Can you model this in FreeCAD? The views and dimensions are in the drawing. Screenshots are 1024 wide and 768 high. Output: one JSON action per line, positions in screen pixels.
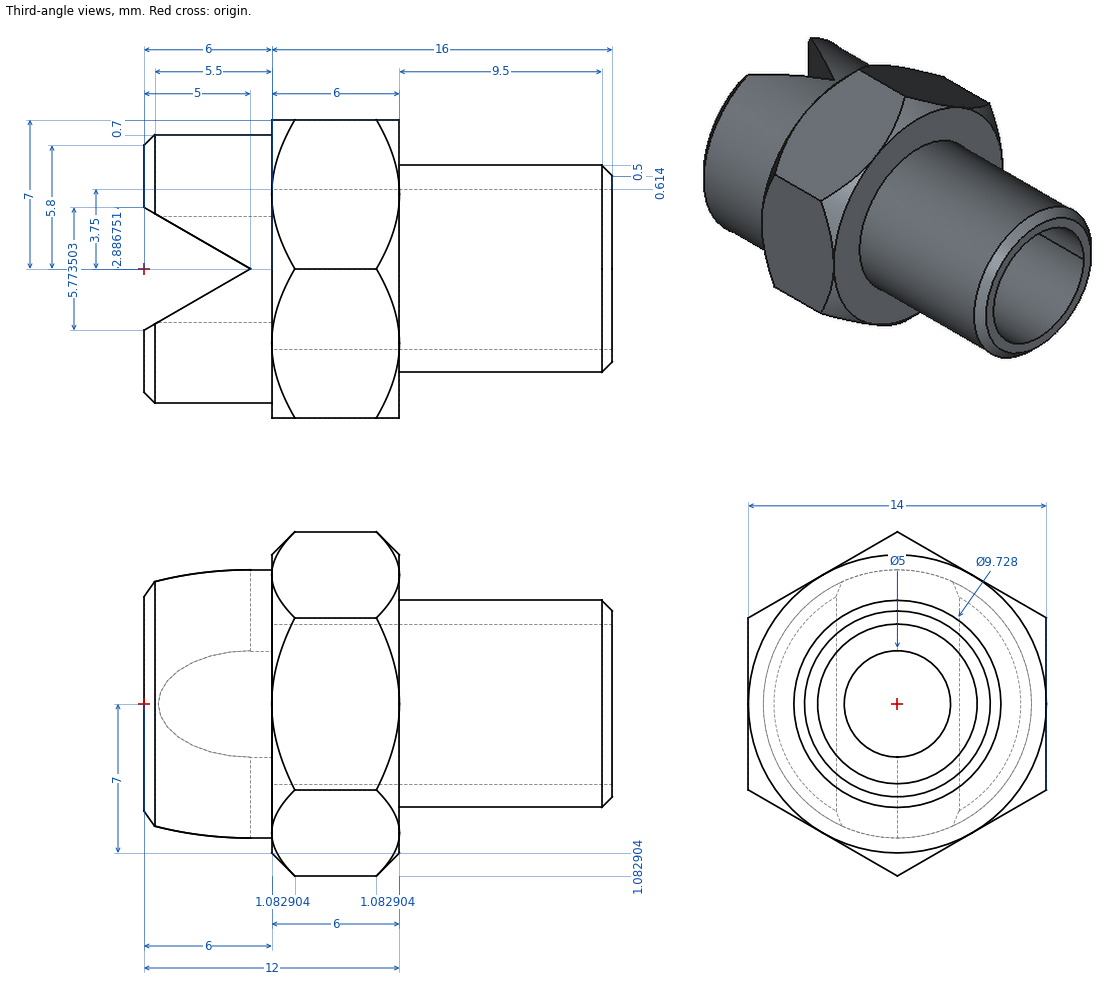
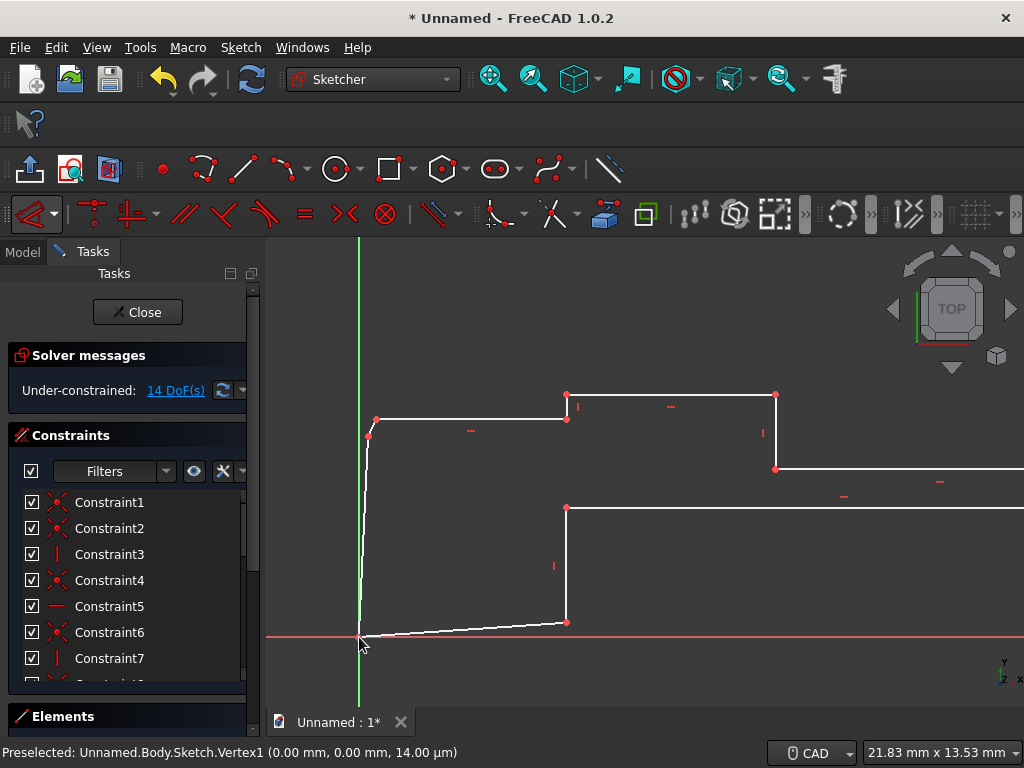
{"action": "scroll", "coordinate": [504, 627], "scroll_direction": "up", "scroll_amount": 2}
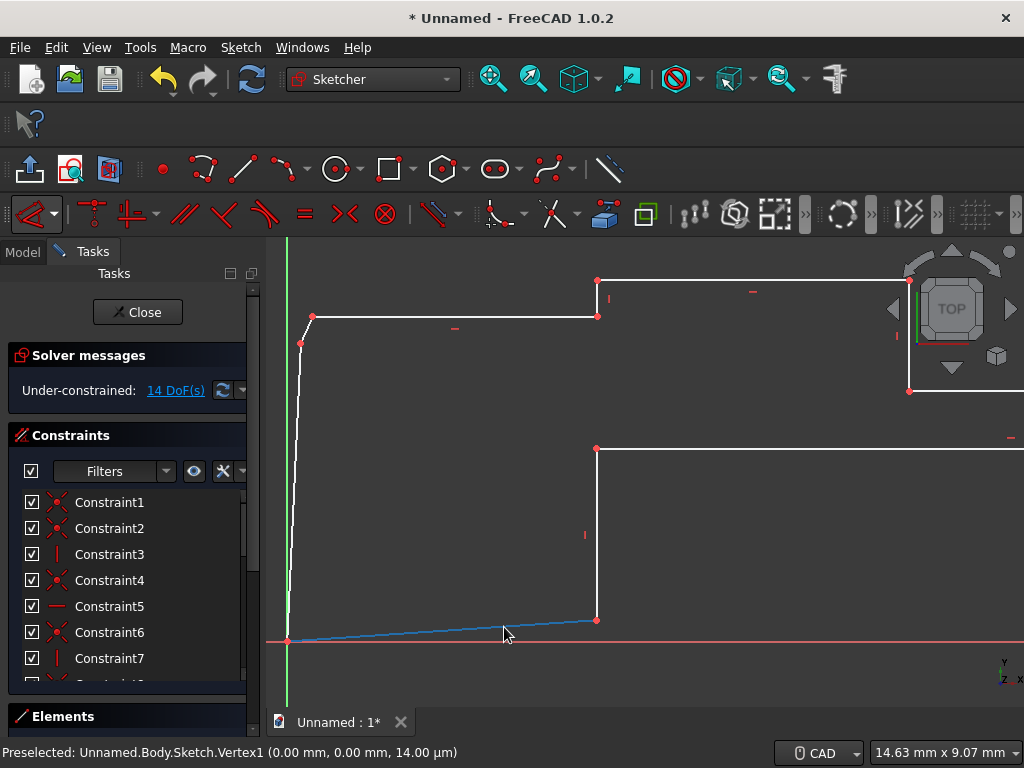
{"action": "left_click", "coordinate": [504, 627]}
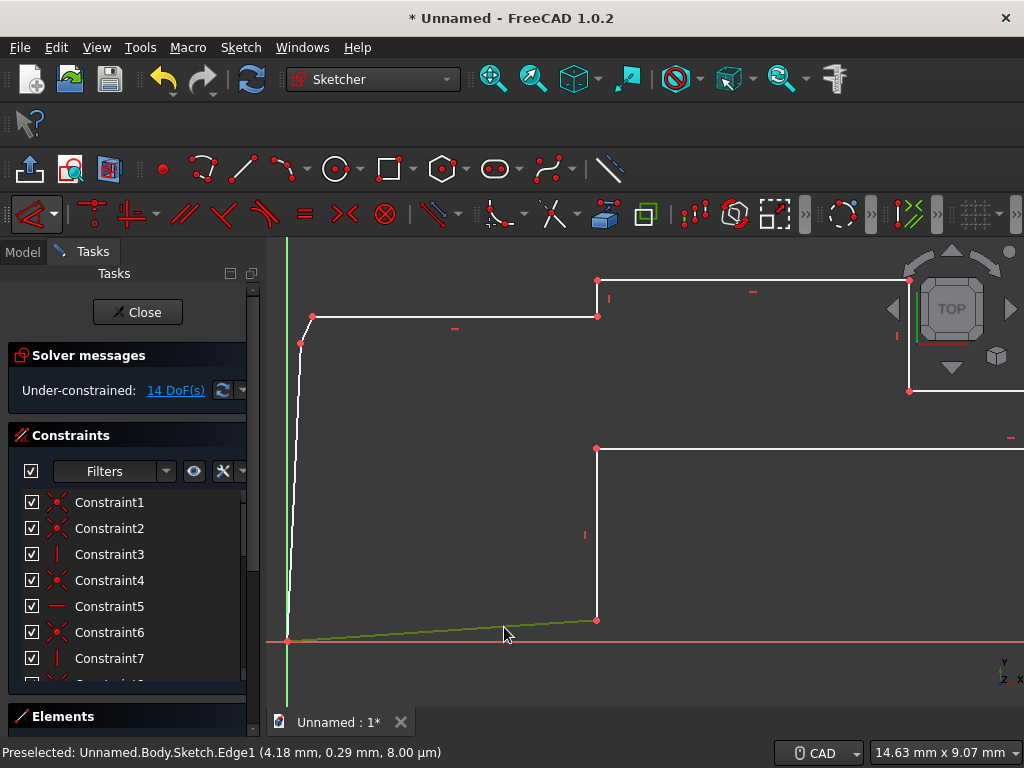
{"action": "left_click", "coordinate": [158, 214]}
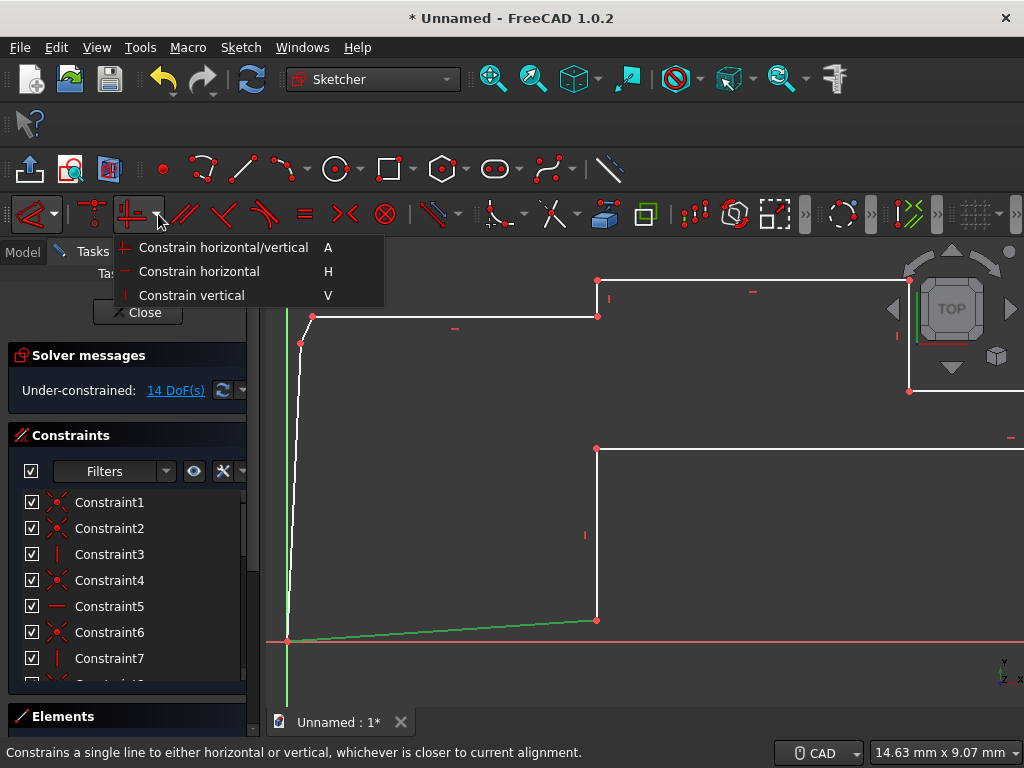
{"action": "left_click", "coordinate": [249, 271]}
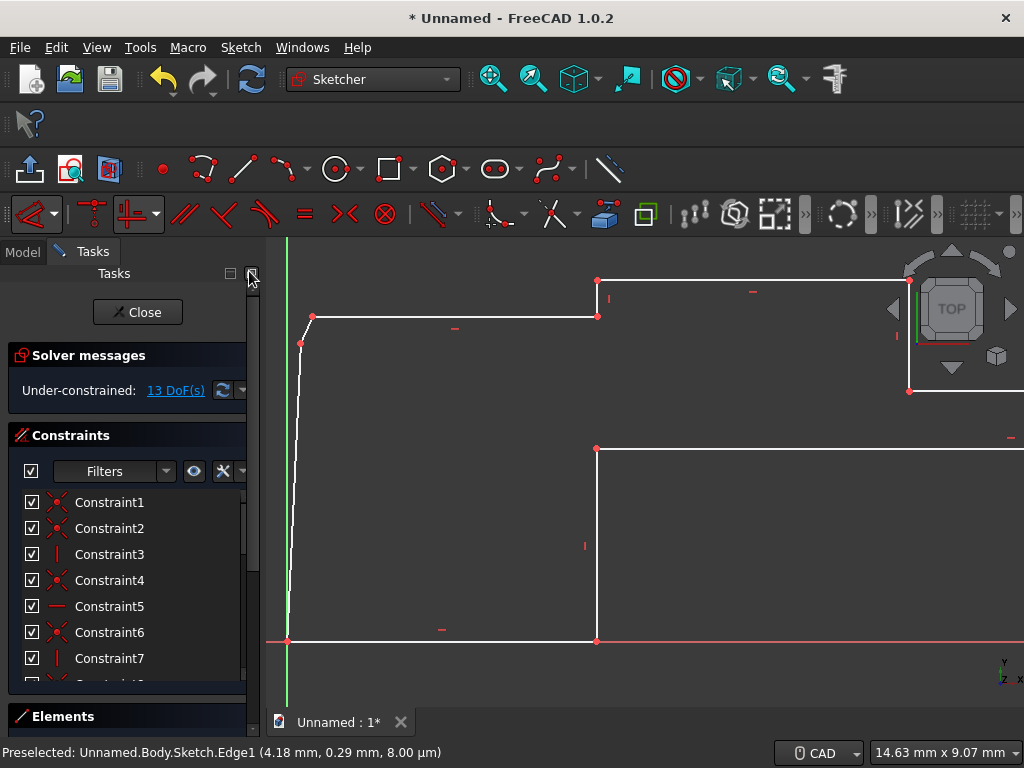
{"action": "scroll", "coordinate": [297, 433], "scroll_direction": "up", "scroll_amount": 2}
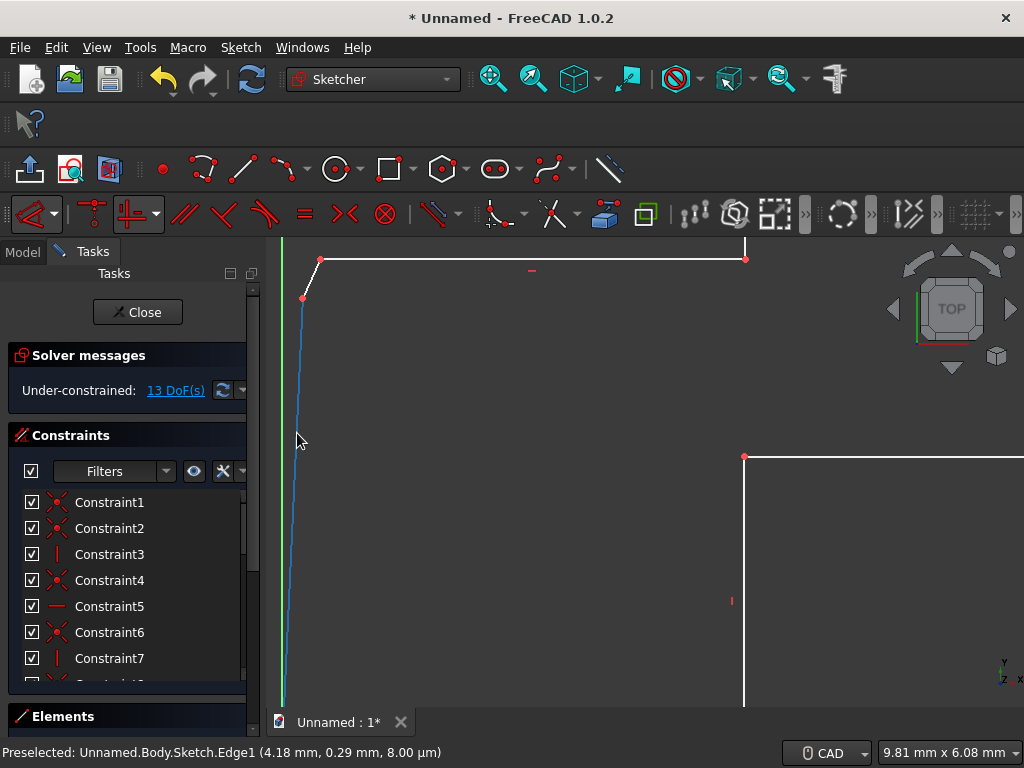
{"action": "left_click", "coordinate": [297, 432]}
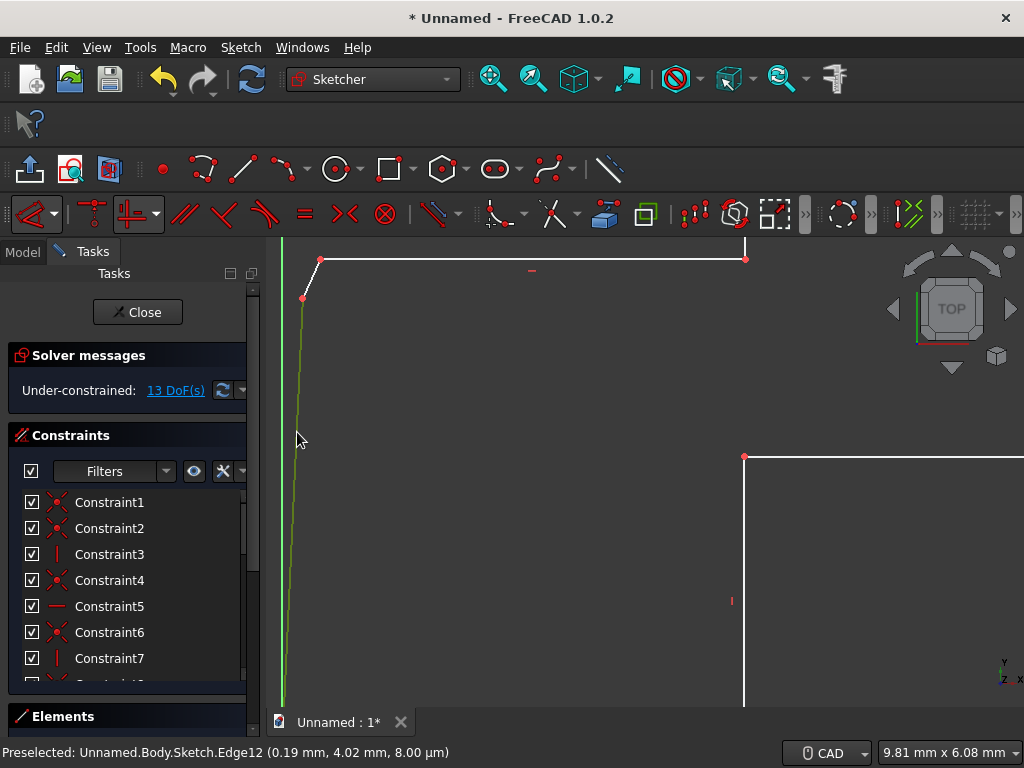
{"action": "key", "text": "v"}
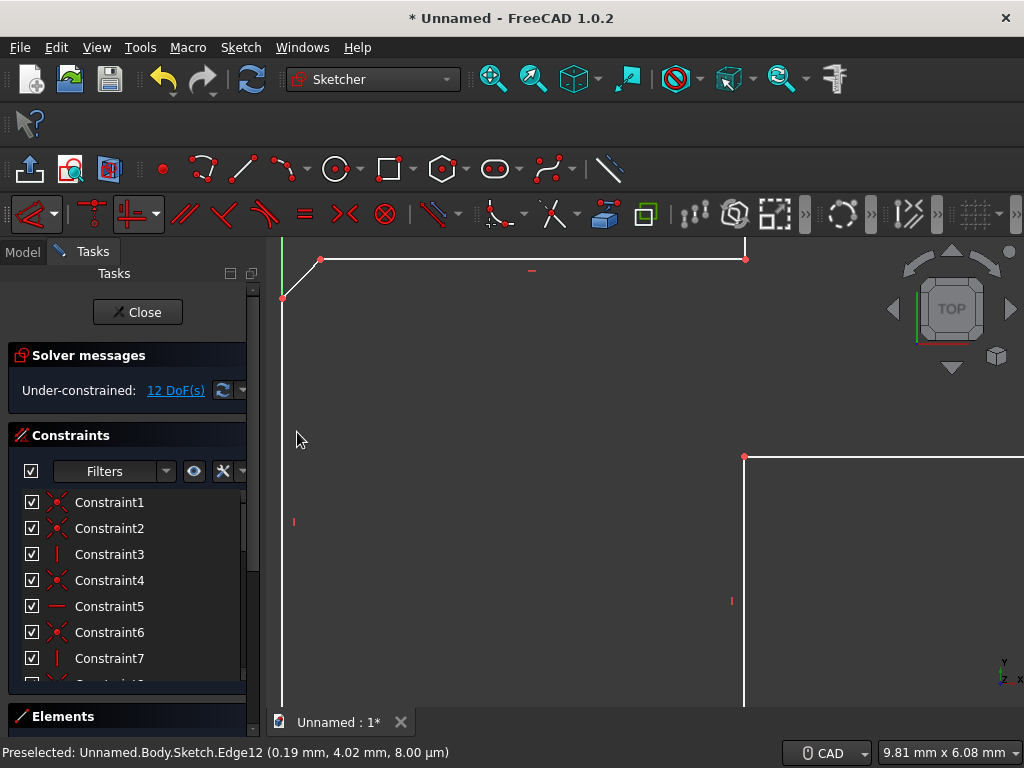
{"action": "left_click", "coordinate": [30, 214]}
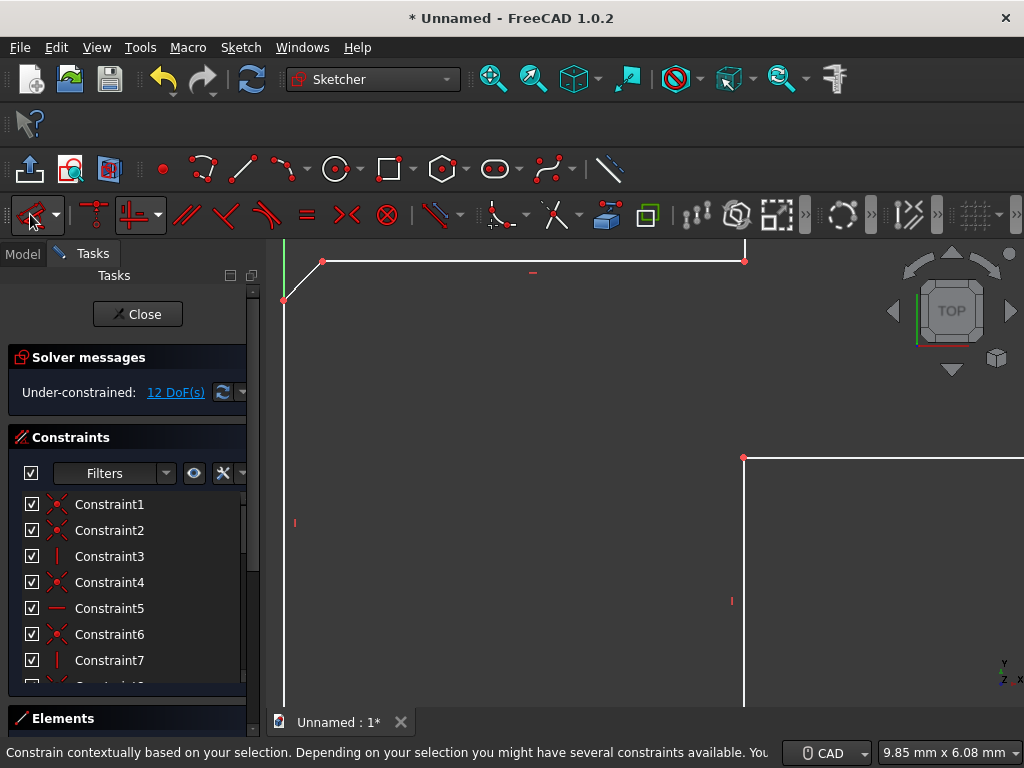
{"action": "scroll", "coordinate": [395, 473], "scroll_direction": "down", "scroll_amount": 7}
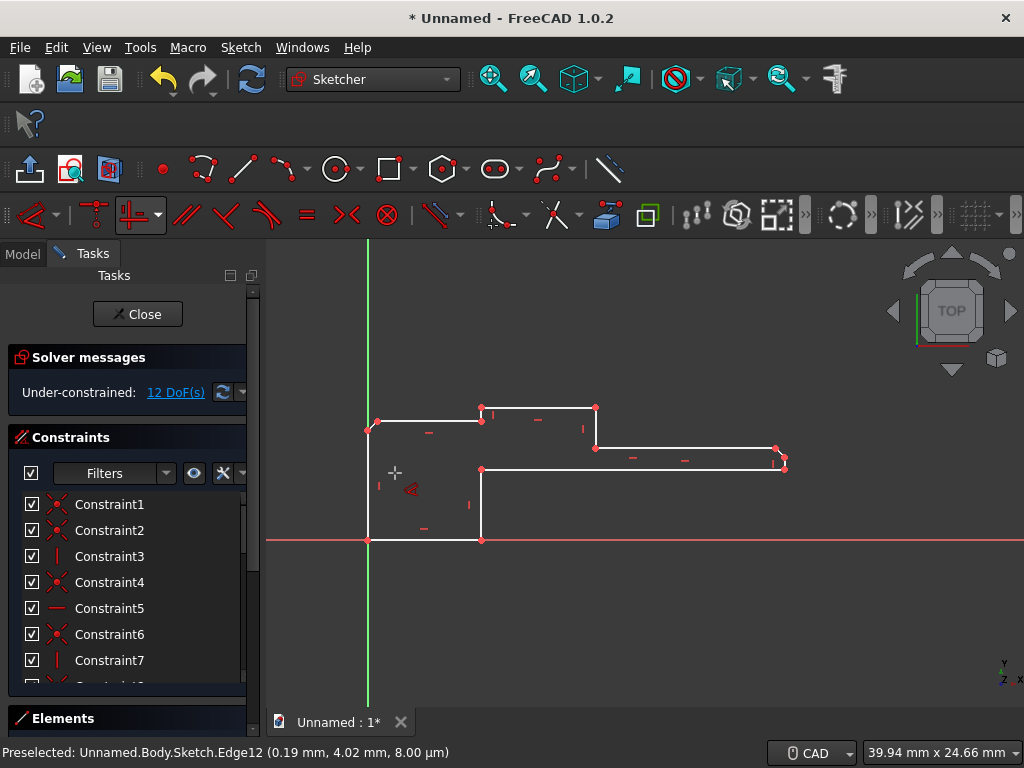
{"action": "left_click", "coordinate": [402, 540]}
{"action": "left_click", "coordinate": [424, 574]}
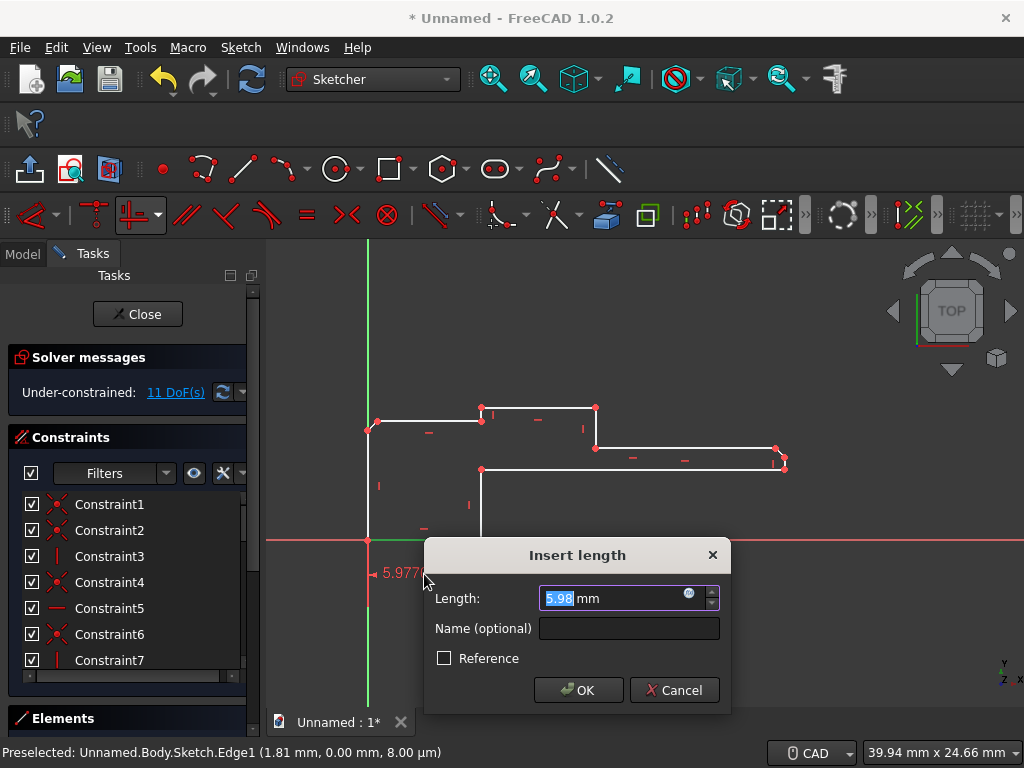
{"action": "type", "text": "6"}
{"action": "key", "text": "Return"}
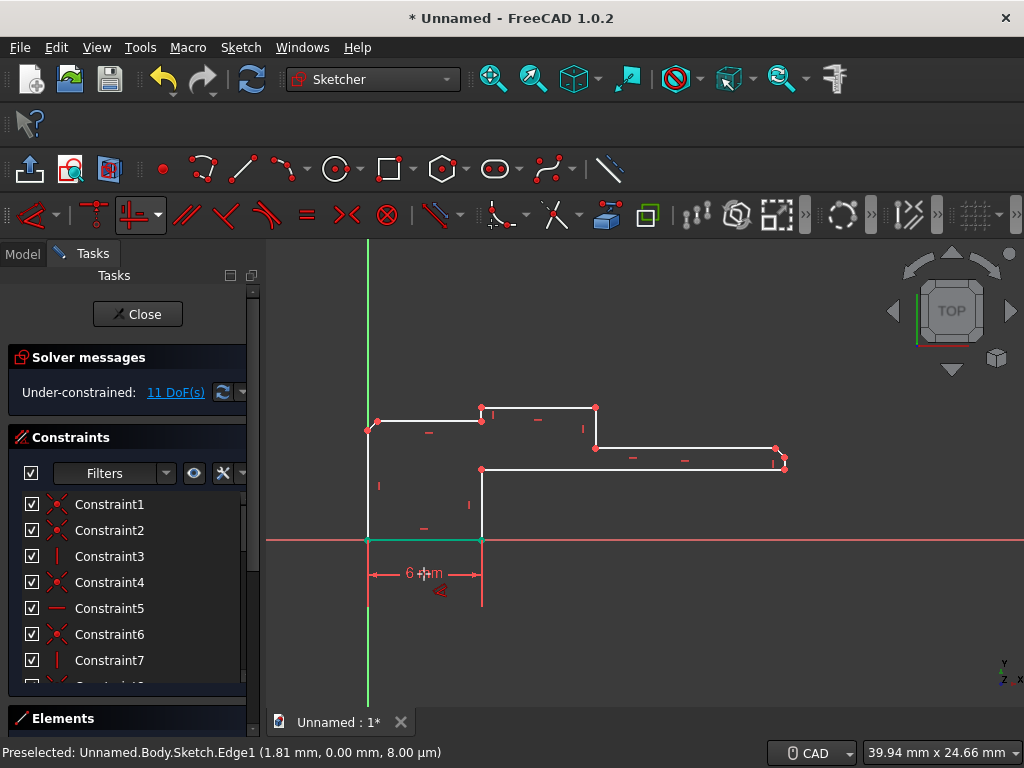
{"action": "left_click", "coordinate": [561, 408]}
{"action": "left_click", "coordinate": [538, 374]}